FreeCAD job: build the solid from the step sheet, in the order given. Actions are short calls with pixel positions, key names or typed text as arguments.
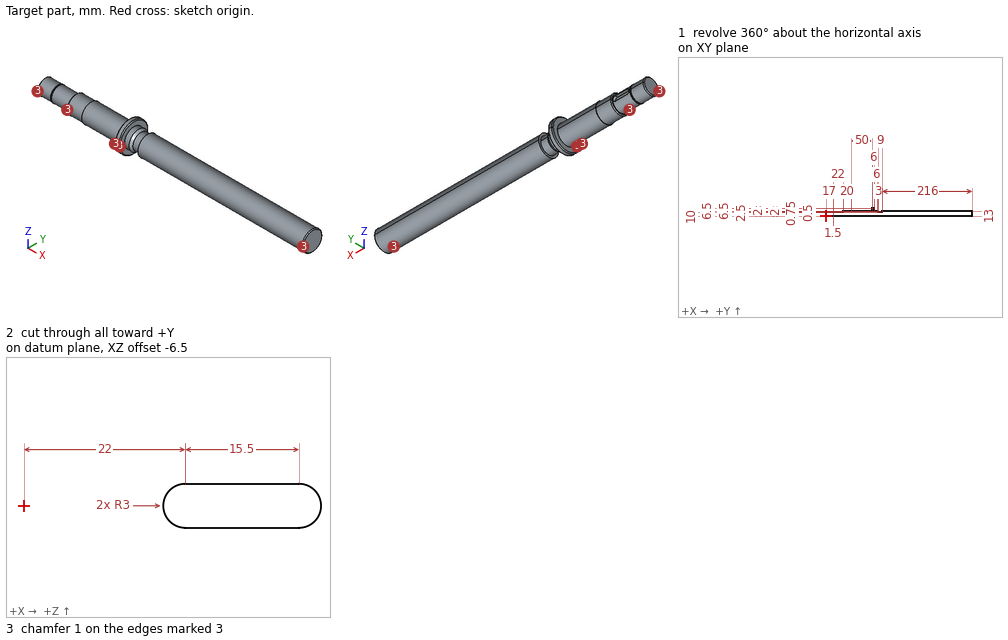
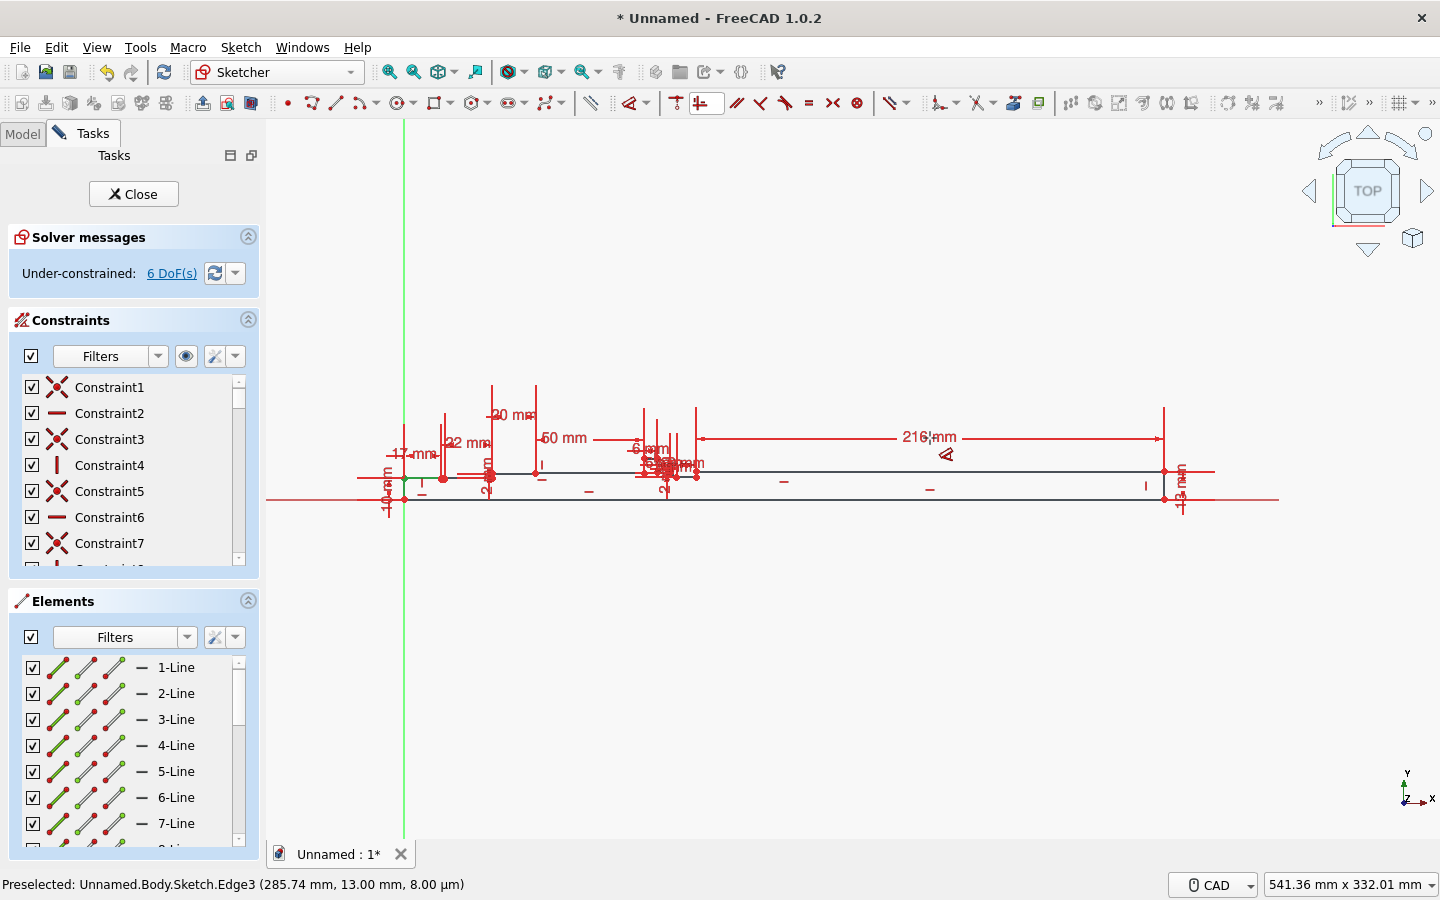
scroll(696, 474, up, 10)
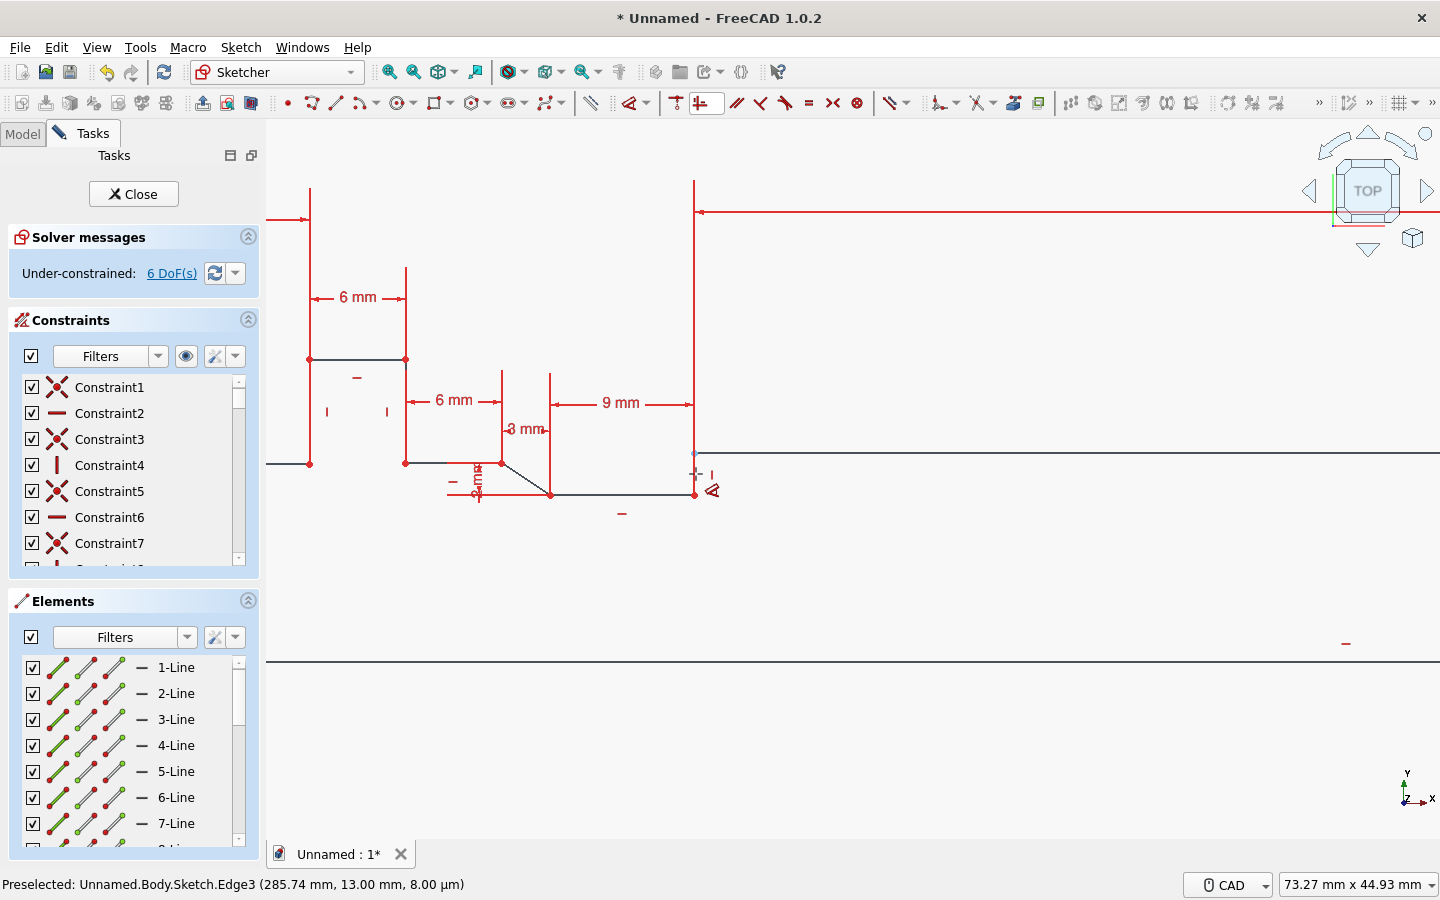
click(694, 474)
click(660, 474)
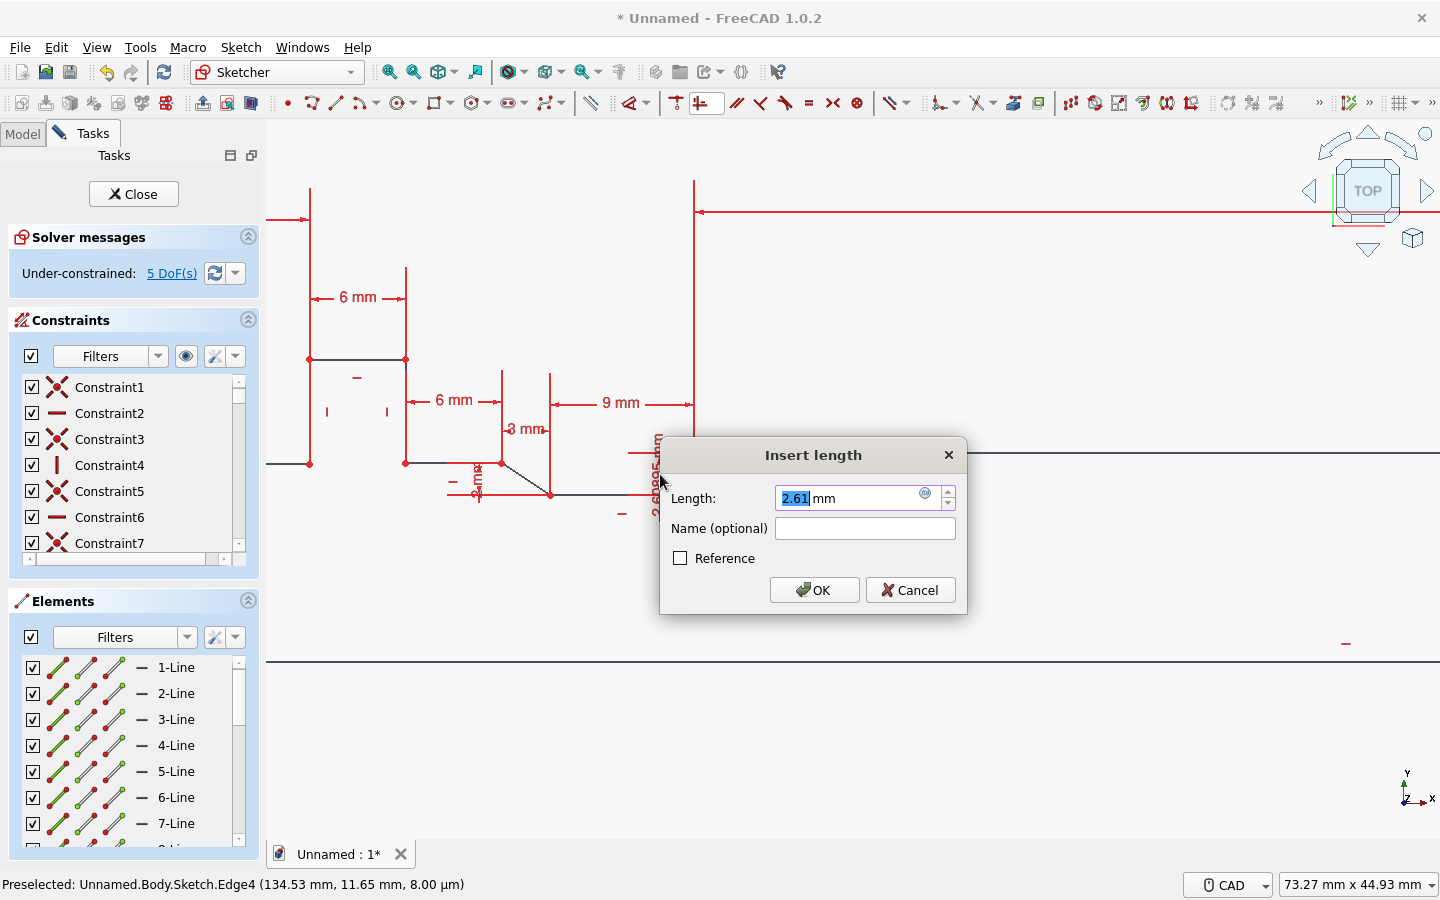
text(2.5)
key(Return)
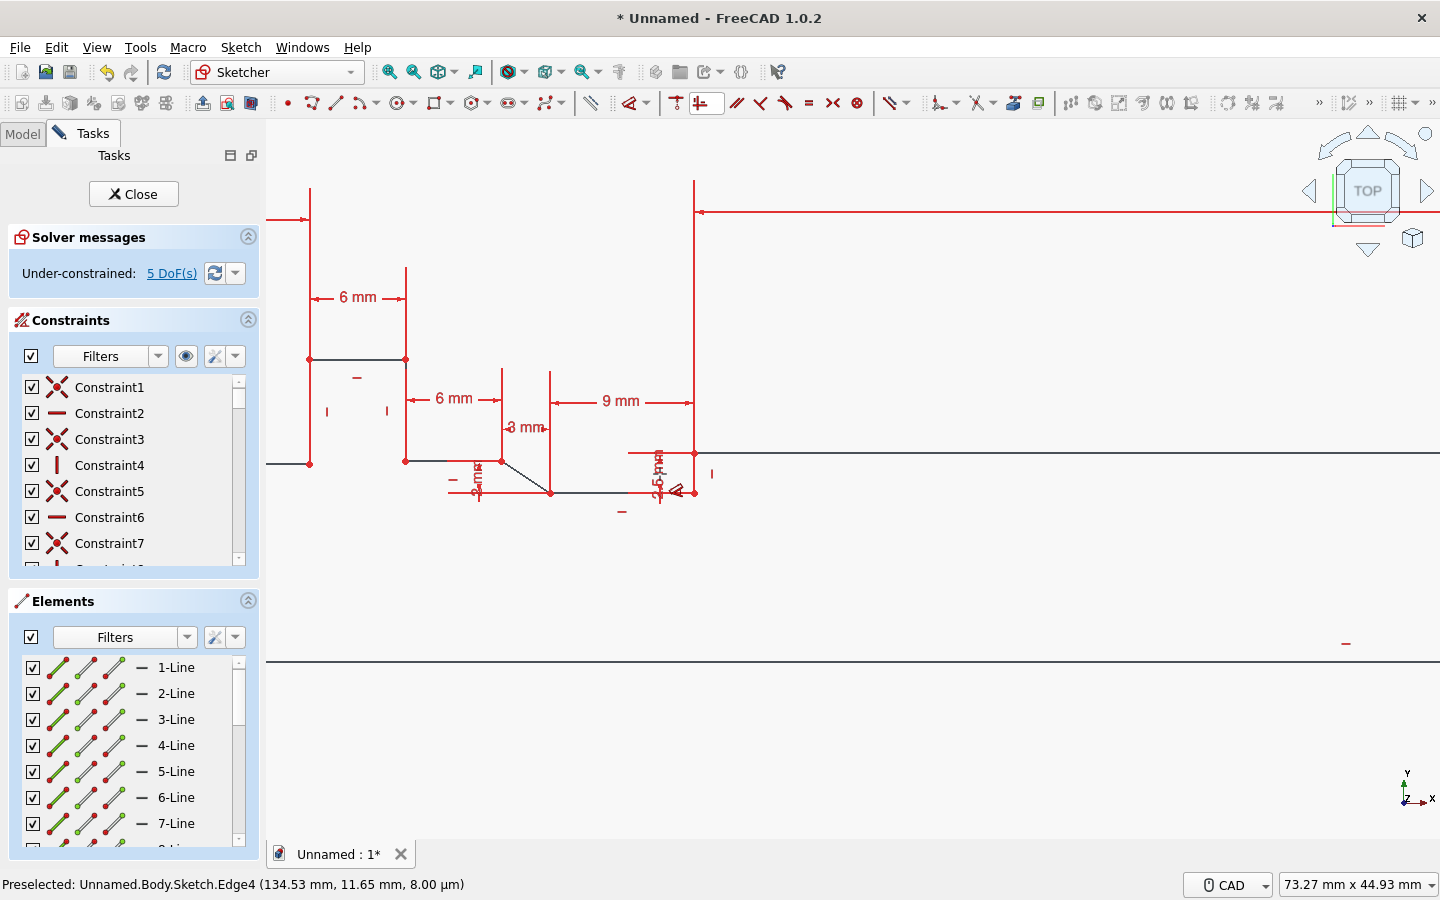
click(406, 431)
click(372, 411)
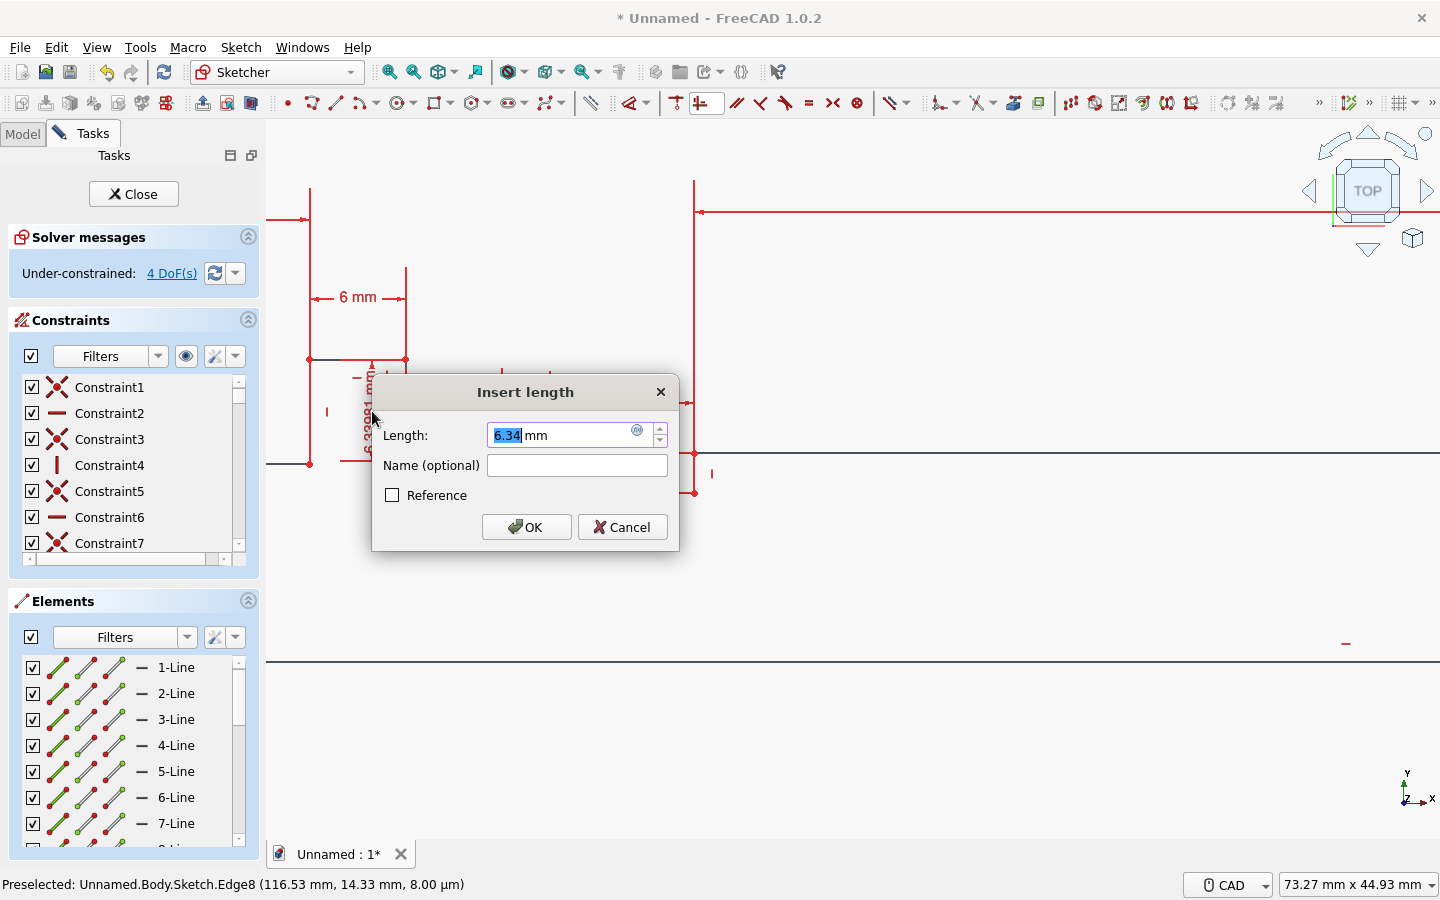
text(6.5)
key(Return)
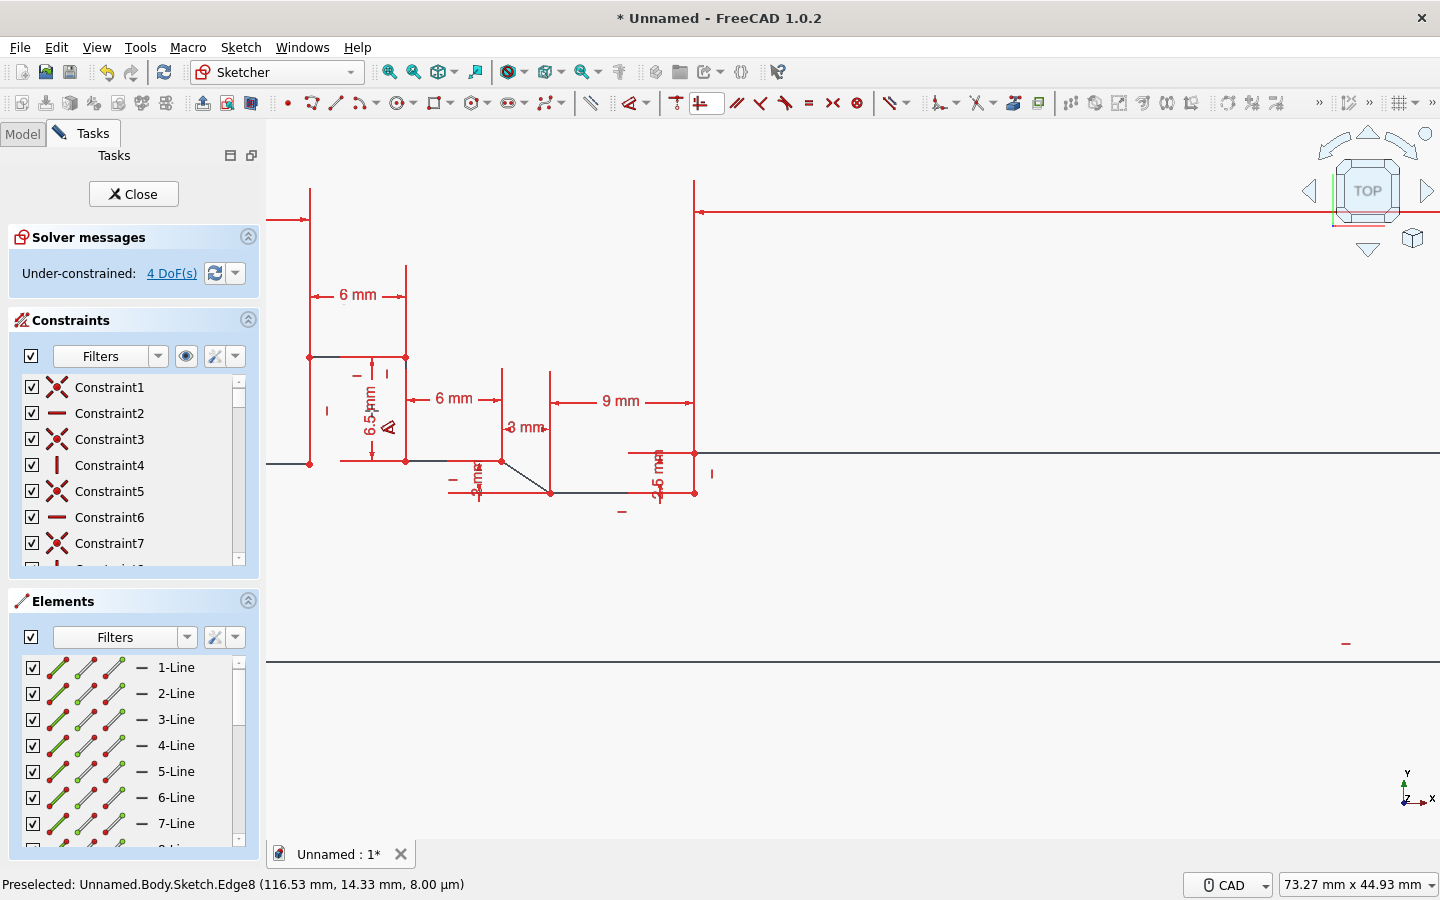
click(310, 389)
click(344, 386)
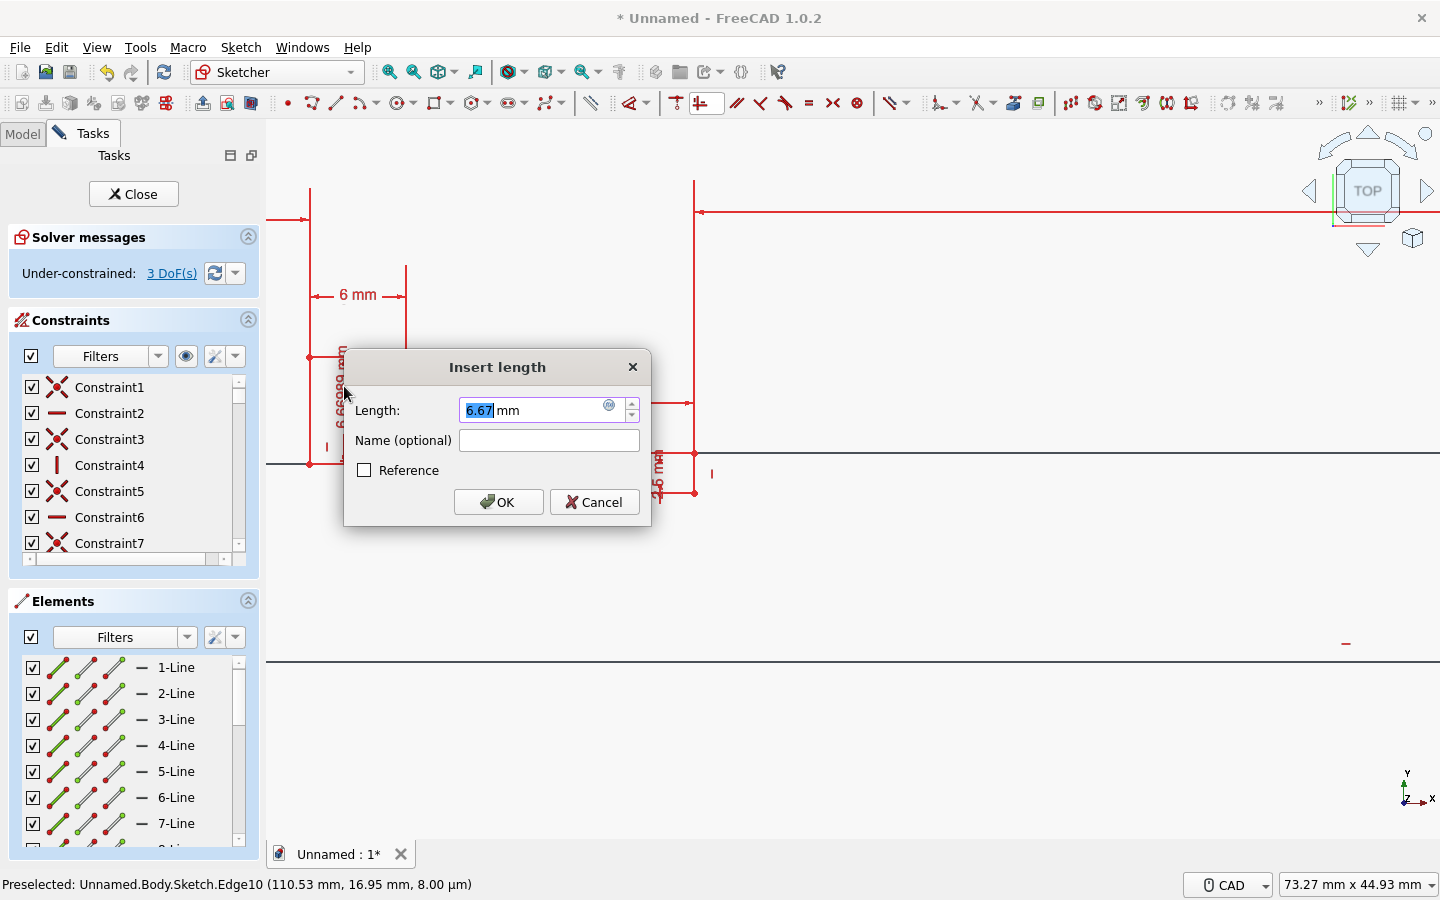
text(6.5)
key(Return)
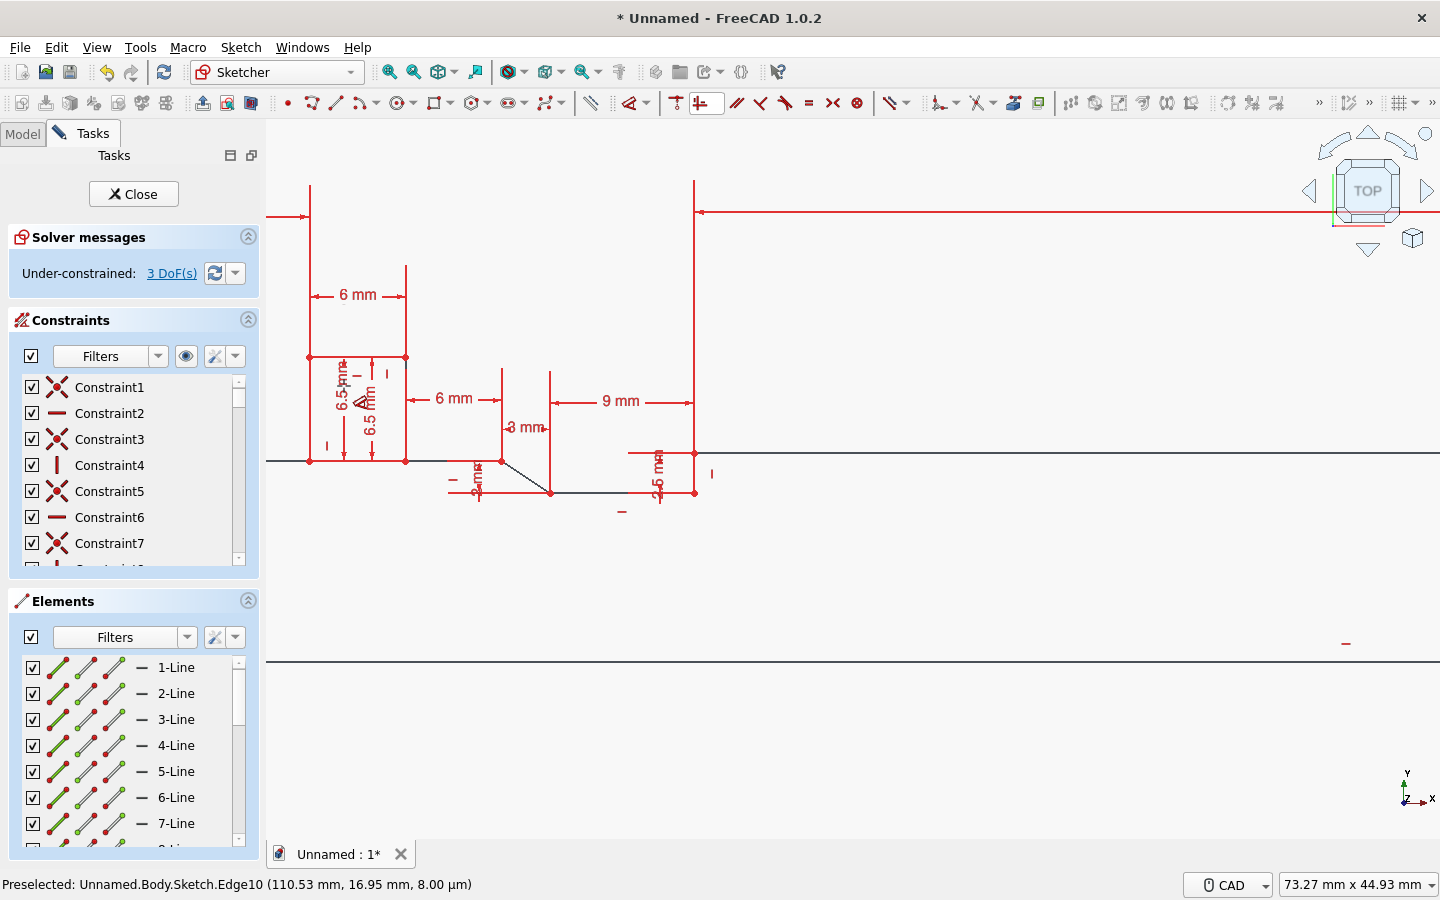
scroll(697, 474, down, 10)